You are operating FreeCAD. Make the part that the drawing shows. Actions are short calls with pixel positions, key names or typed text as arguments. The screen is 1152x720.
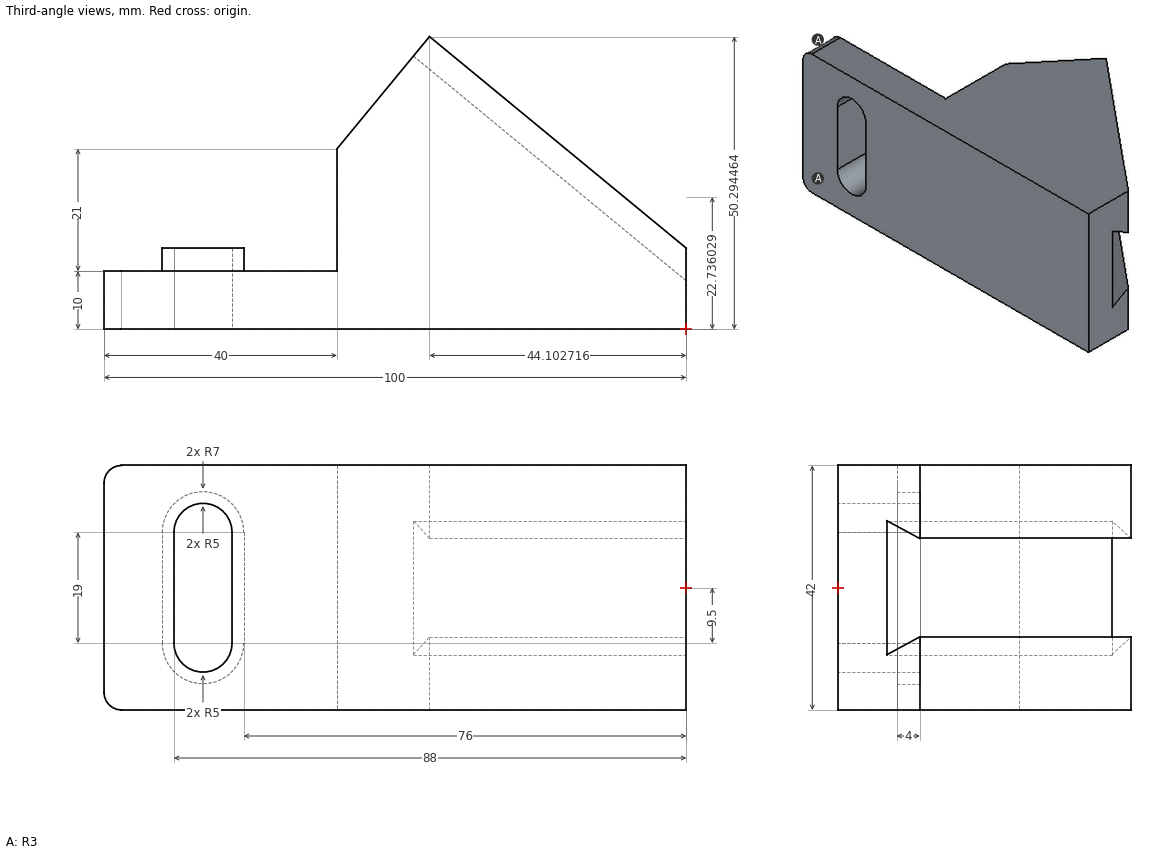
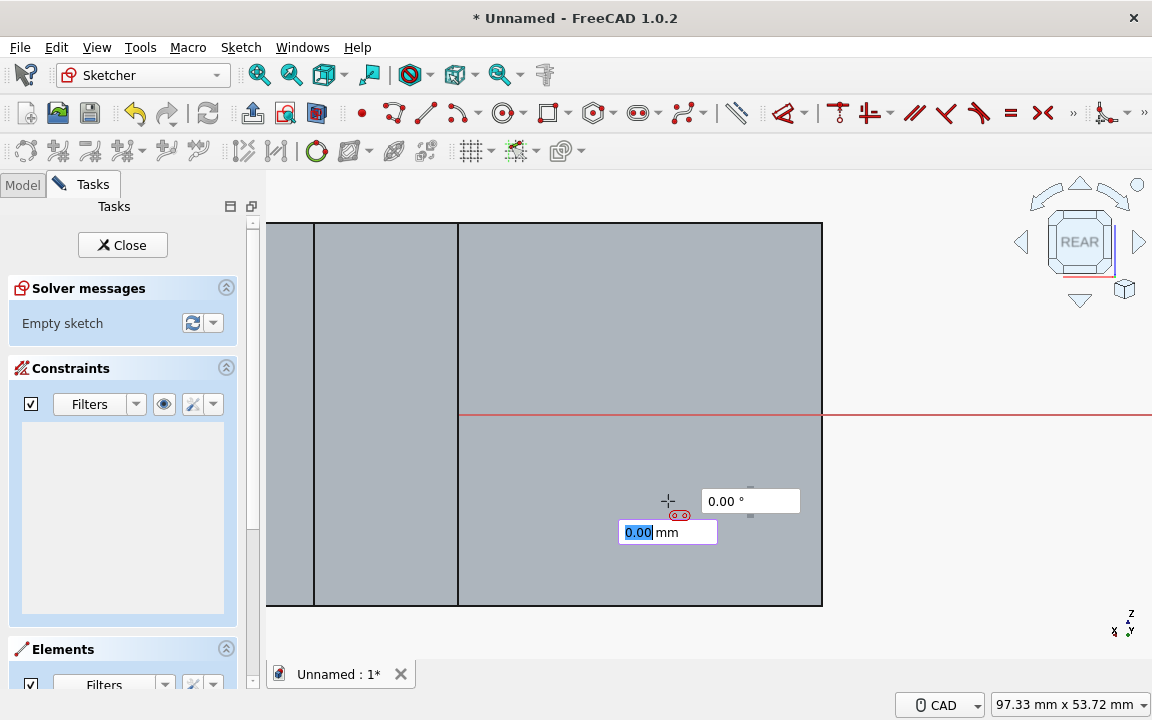
click(668, 328)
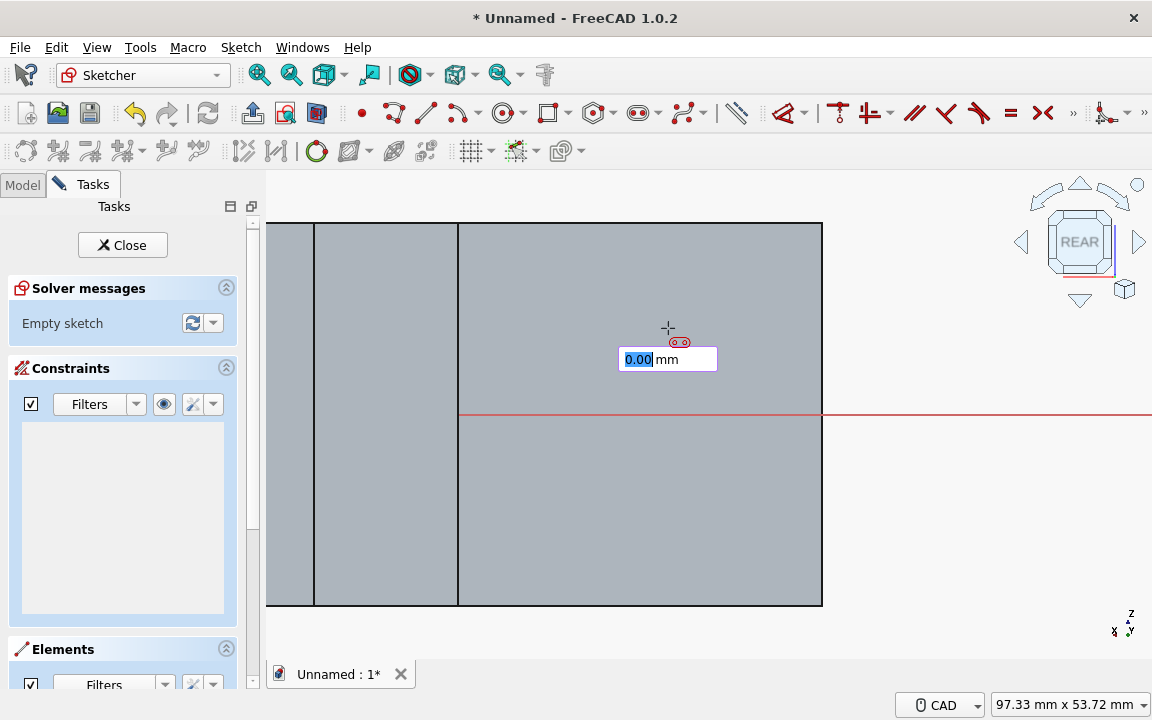
click(731, 440)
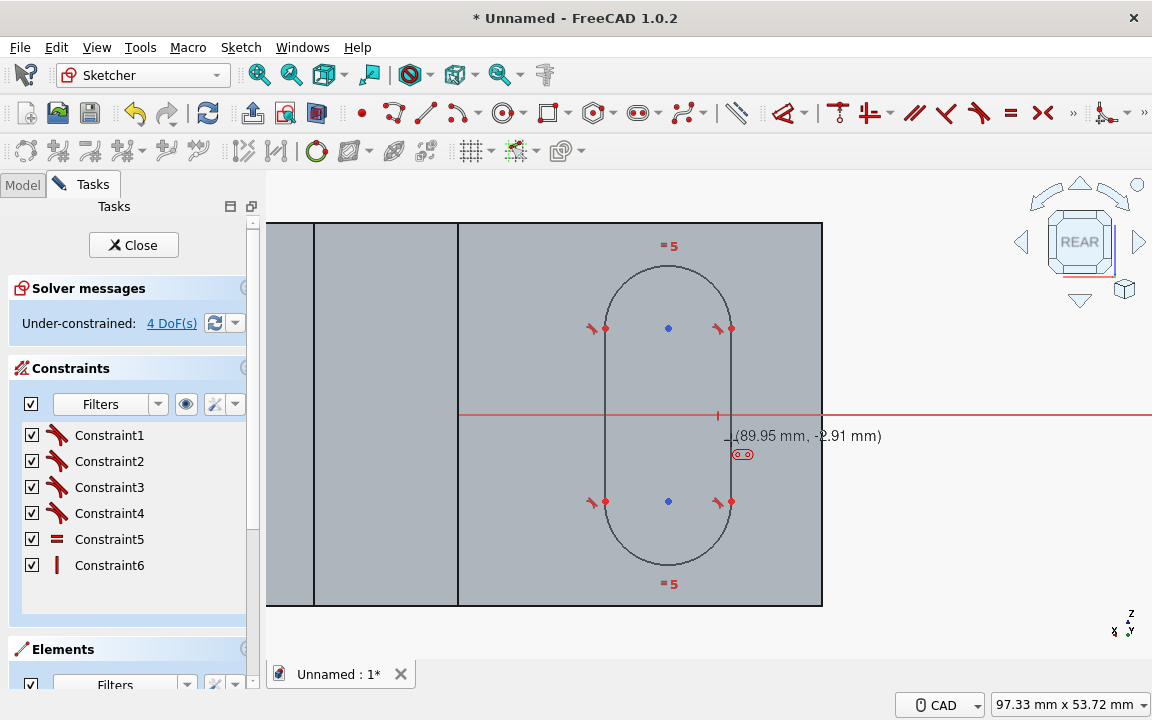
click(668, 502)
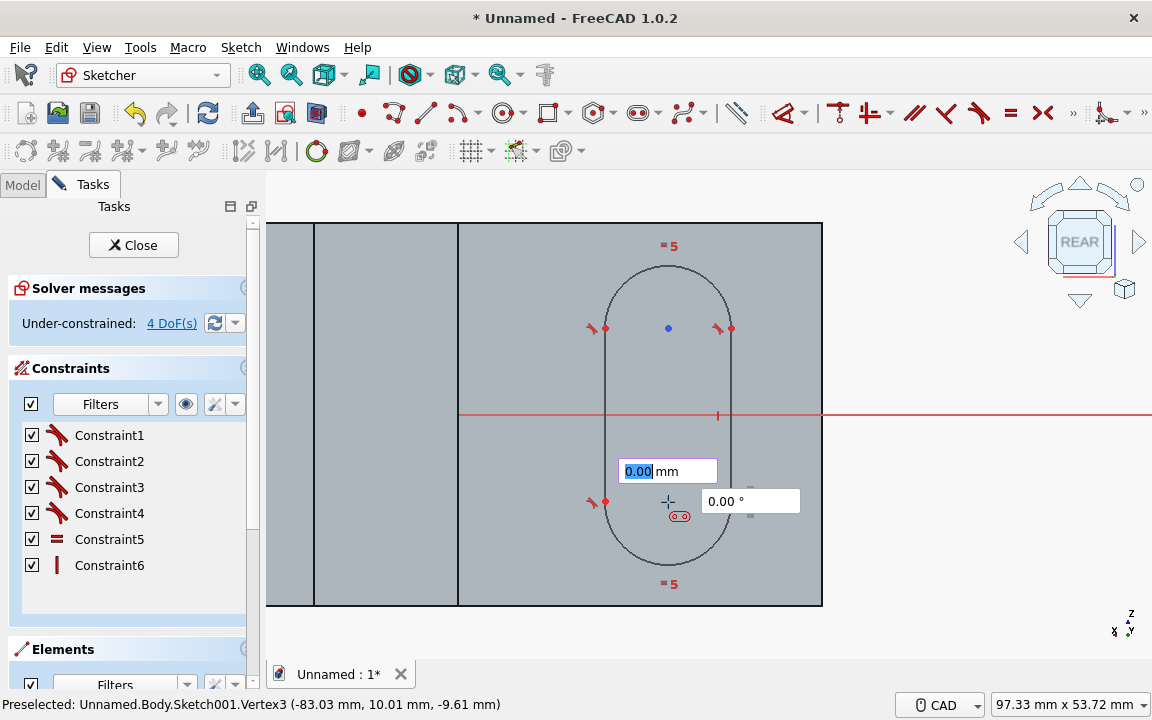
click(668, 329)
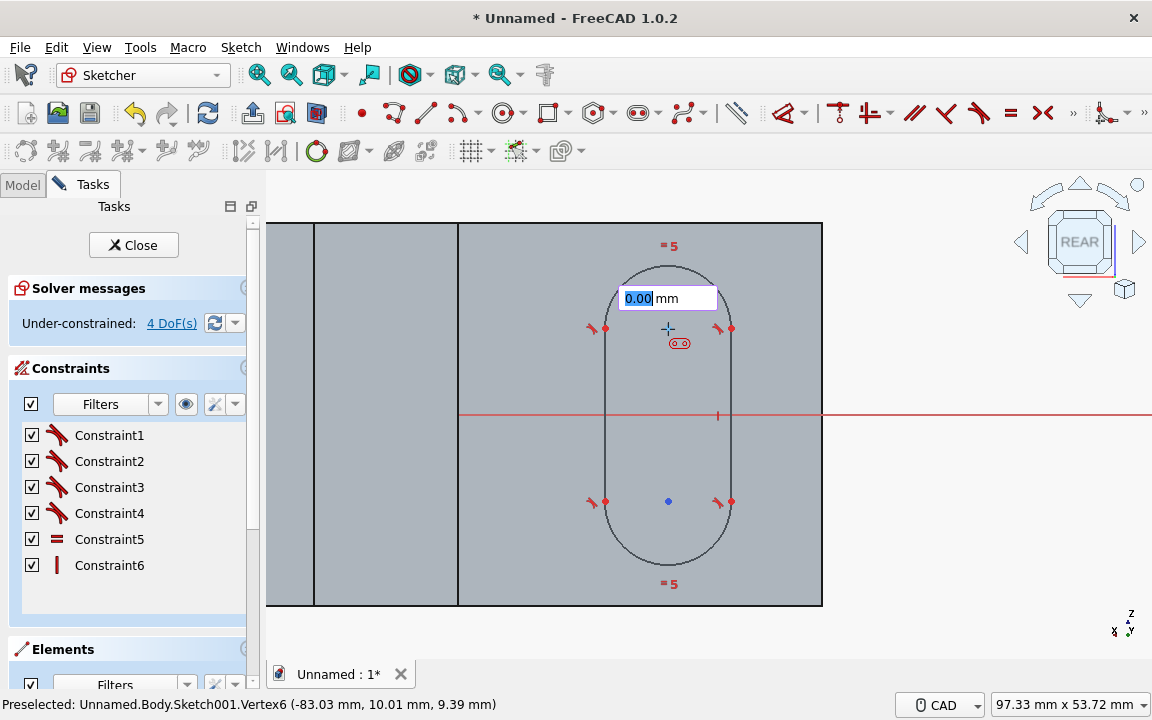
click(713, 389)
key(Escape)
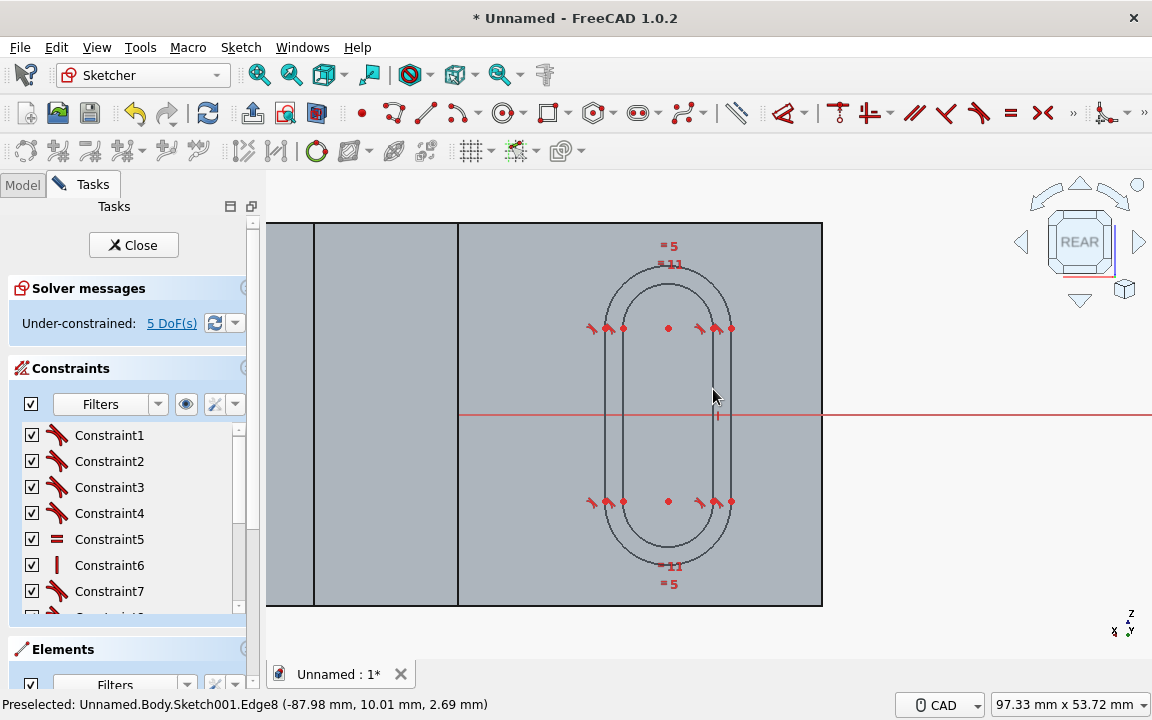
key(d)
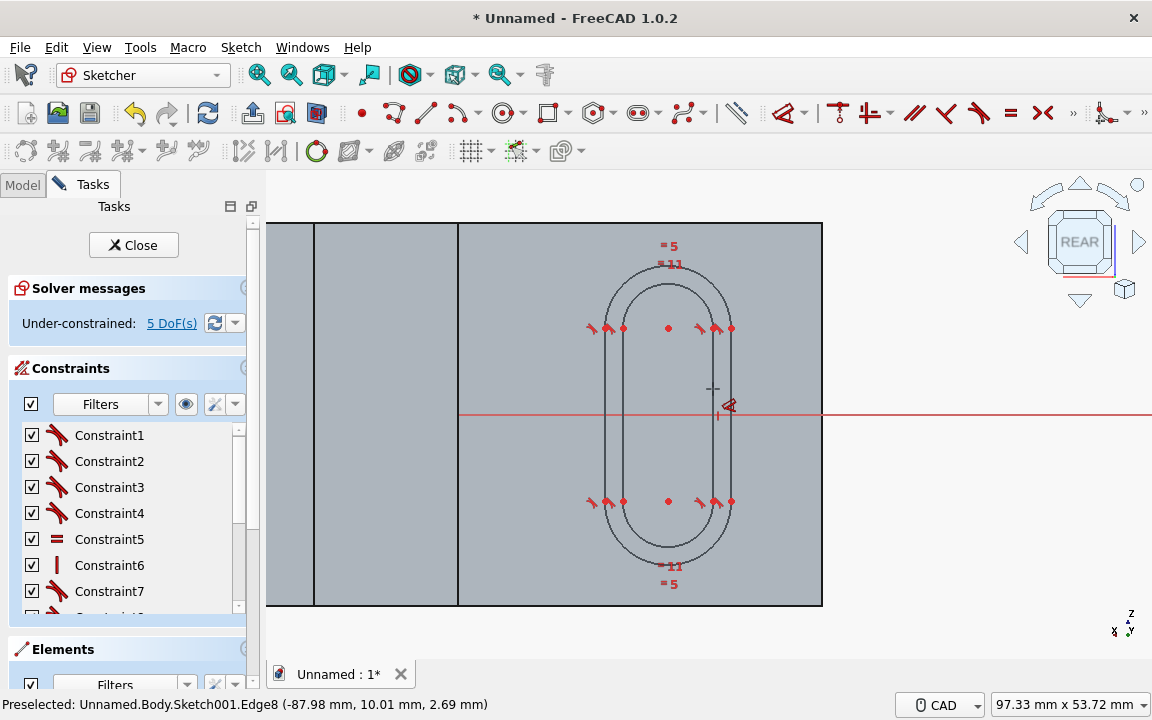
click(631, 553)
click(612, 579)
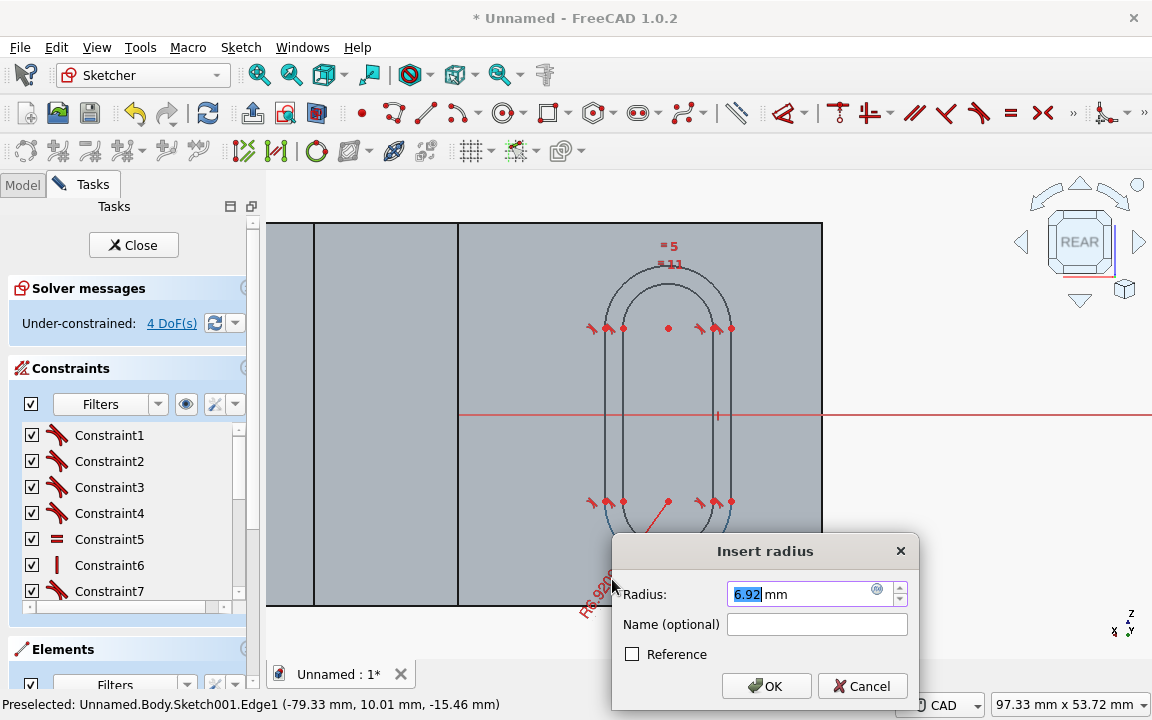
text(7)
key(Return)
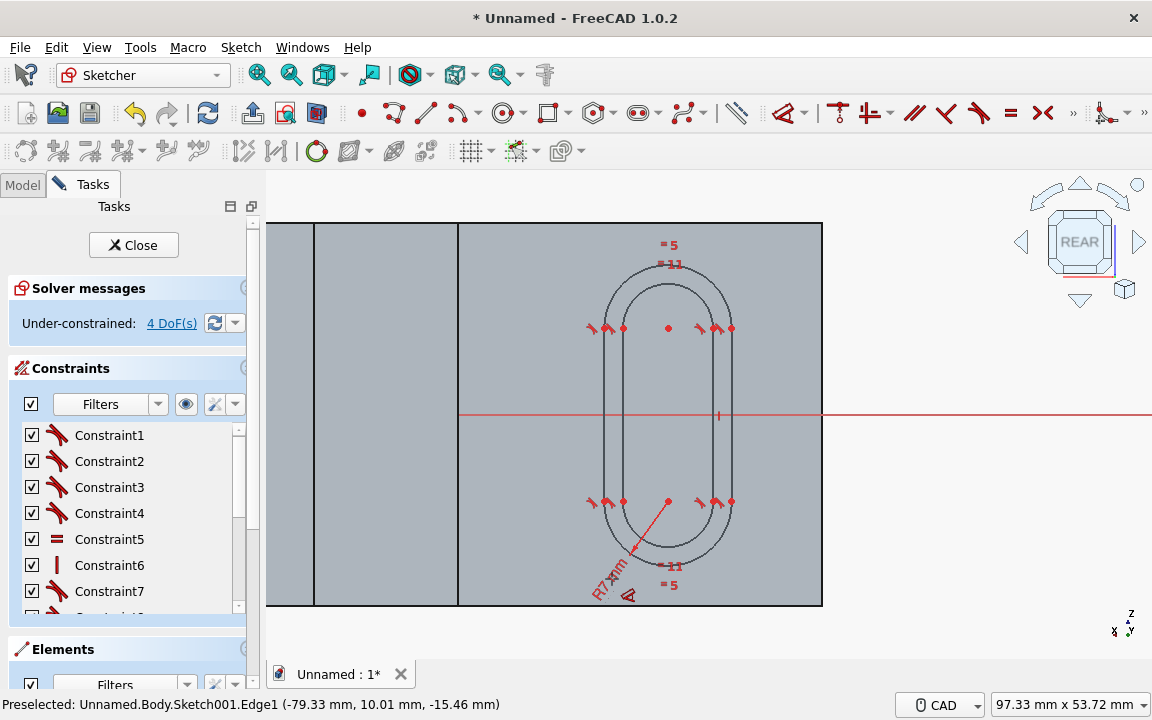
click(642, 538)
click(578, 545)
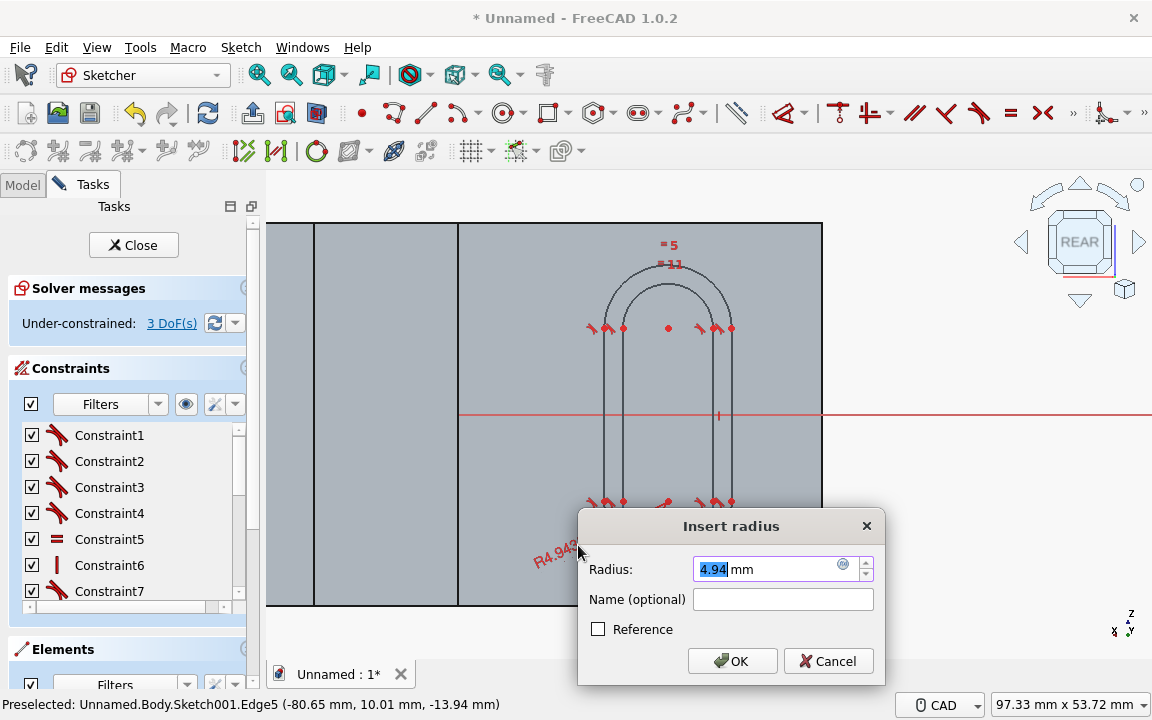
text(5)
key(Return)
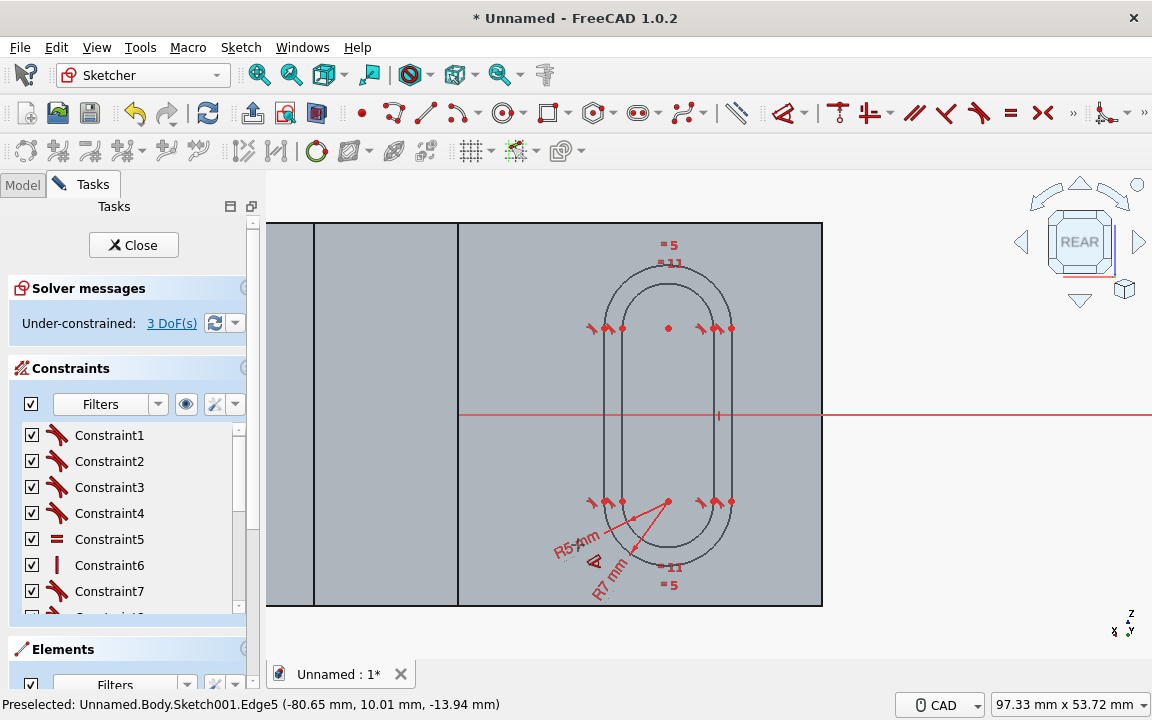
click(604, 450)
click(570, 376)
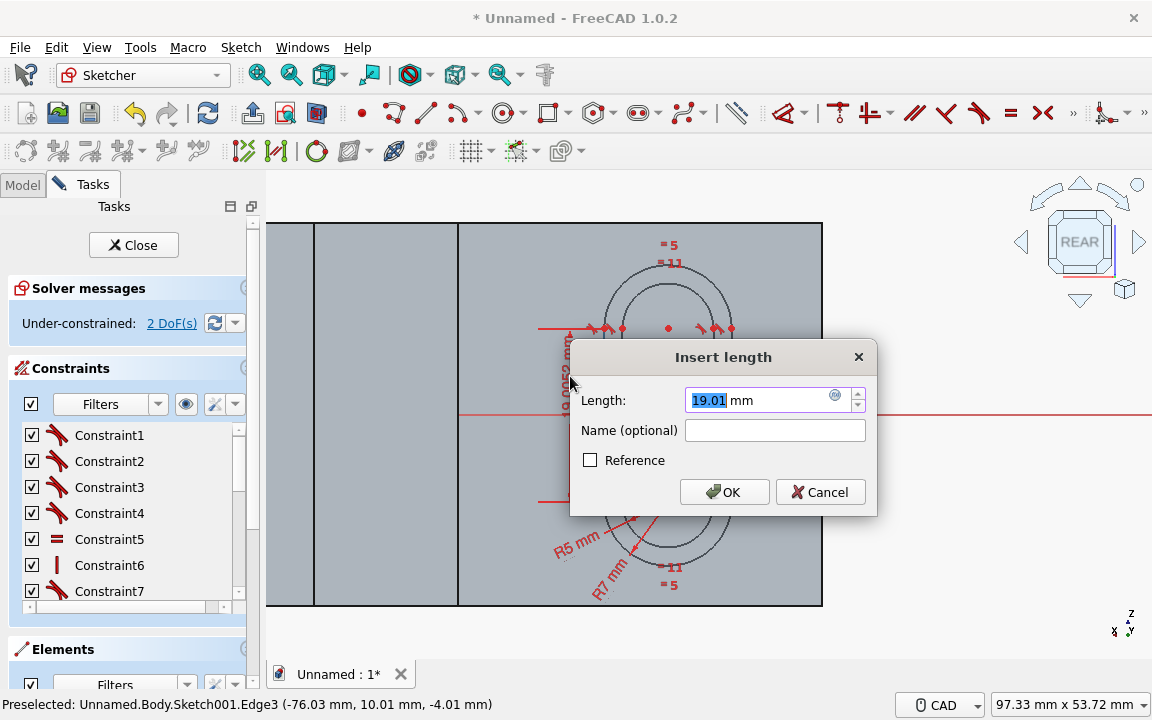
text(19)
key(Return)